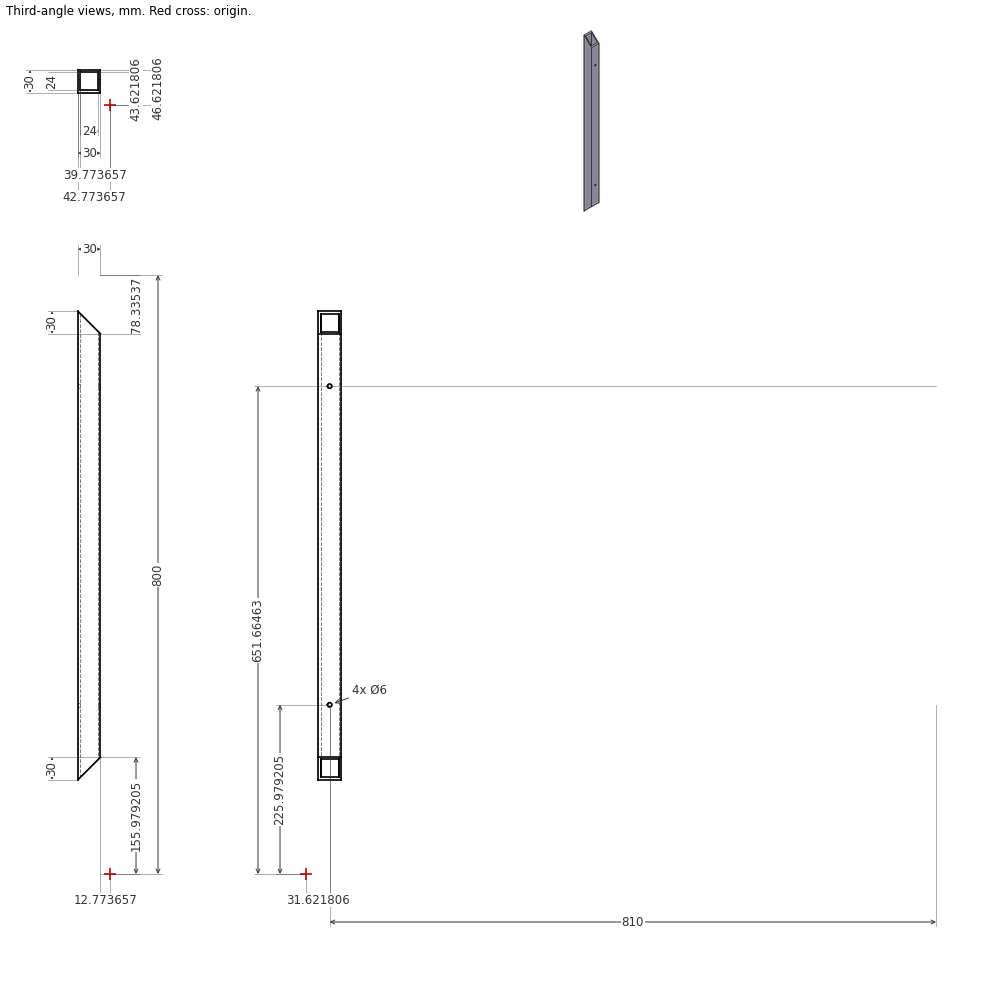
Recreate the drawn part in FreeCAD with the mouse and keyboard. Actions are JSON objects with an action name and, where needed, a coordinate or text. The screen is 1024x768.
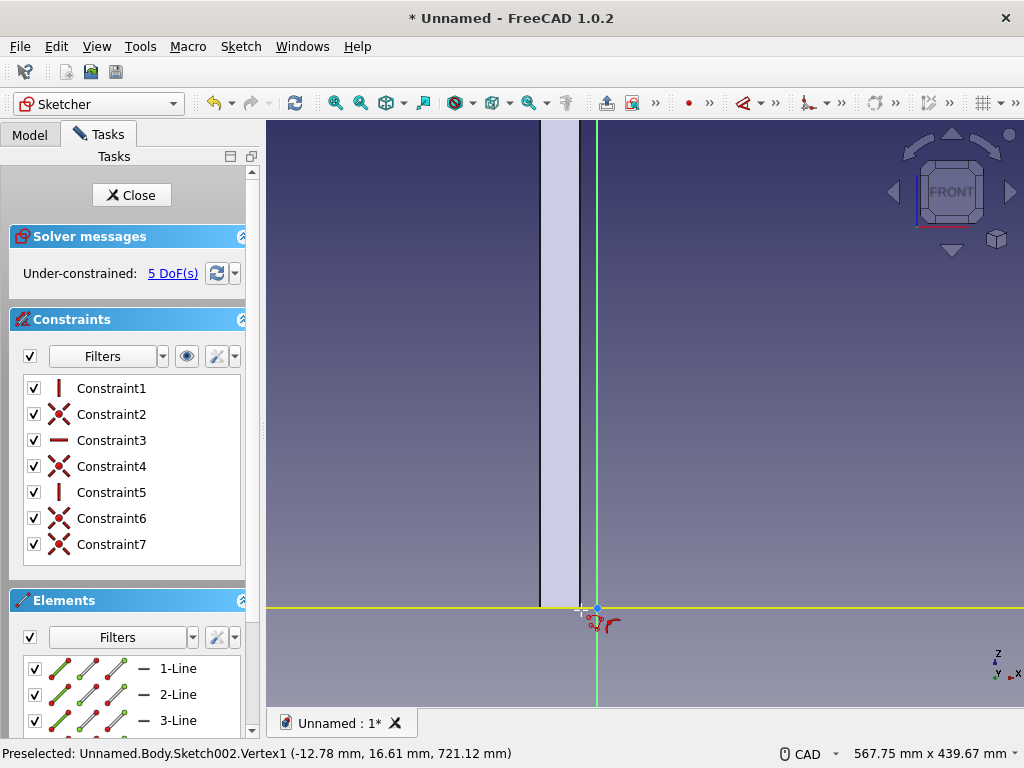
{"action": "left_click", "coordinate": [580, 608]}
{"action": "left_click", "coordinate": [580, 400]}
{"action": "left_click", "coordinate": [540, 440]}
{"action": "left_click", "coordinate": [540, 599]}
{"action": "left_click", "coordinate": [580, 608]}
{"action": "key", "text": "Escape"}
{"action": "key", "text": "Escape"}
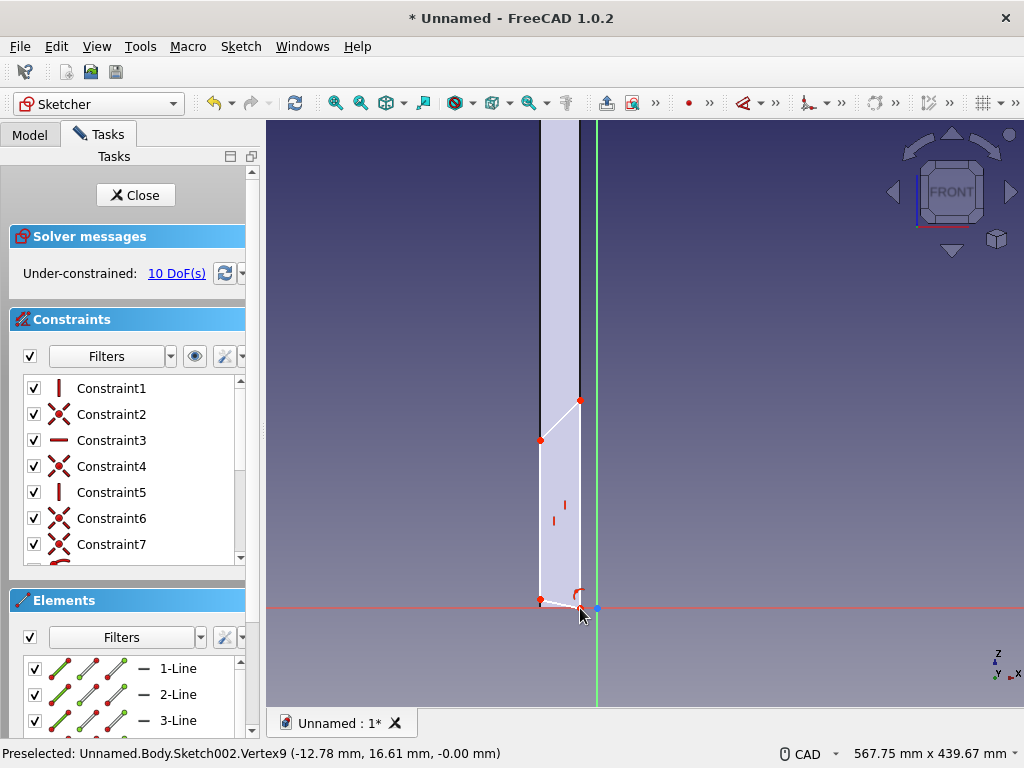
{"action": "left_click", "coordinate": [568, 606]}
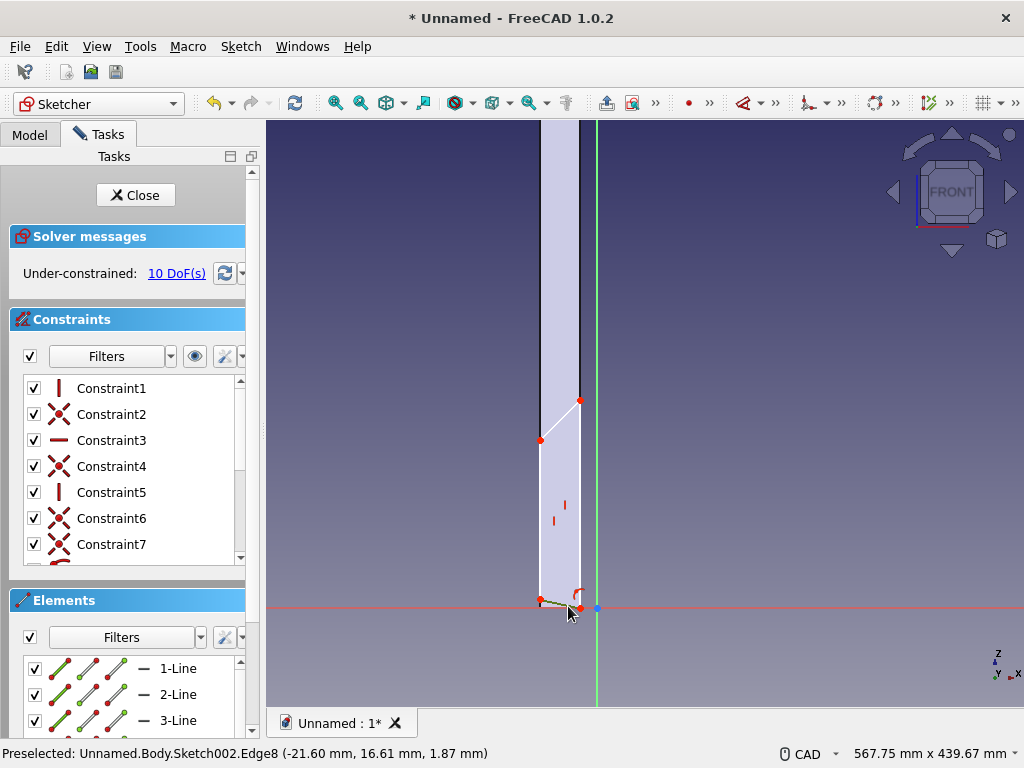
{"action": "key", "text": "h"}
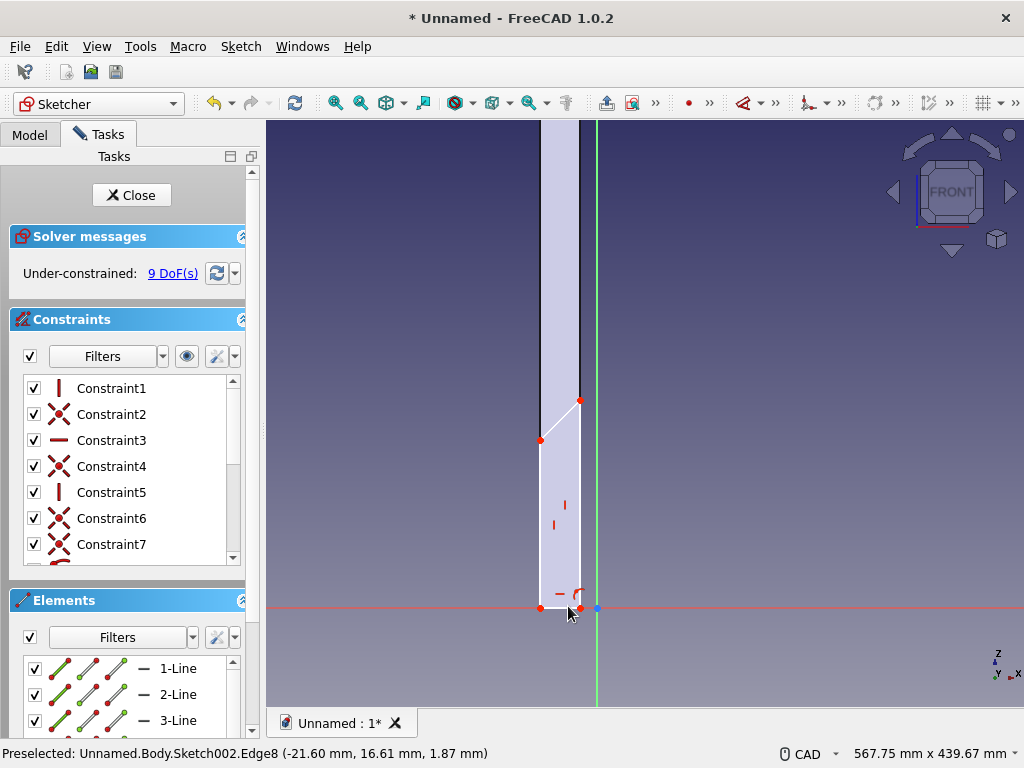
{"action": "key", "text": "d"}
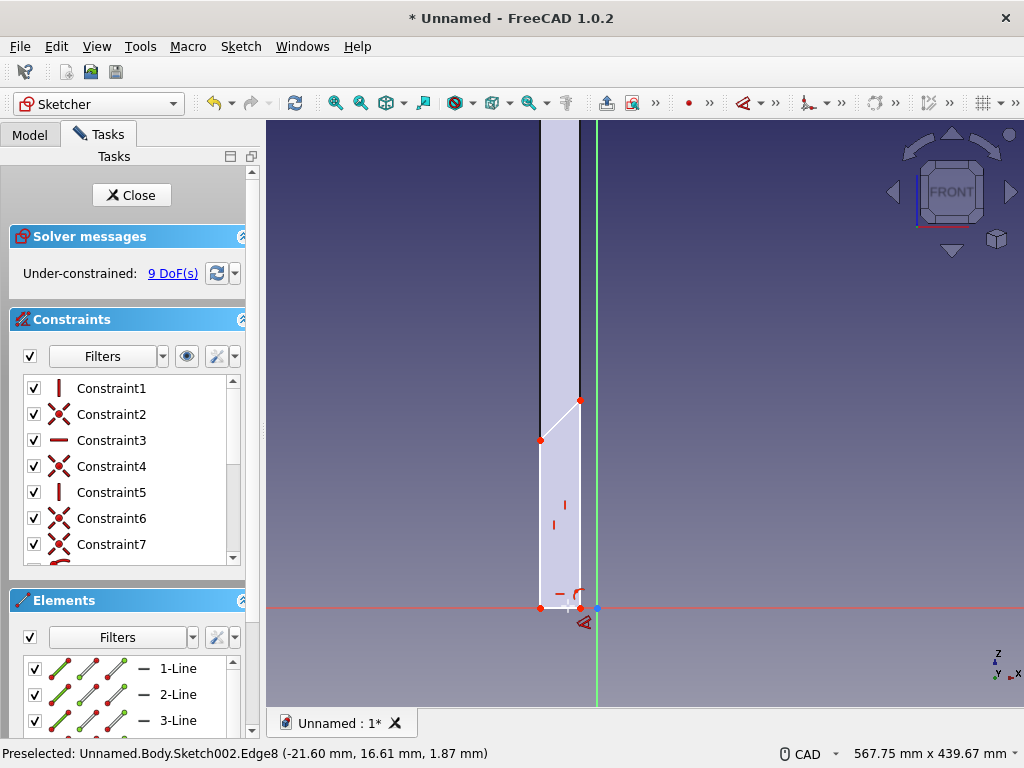
{"action": "scroll", "coordinate": [581, 611], "scroll_direction": "down", "scroll_amount": 5}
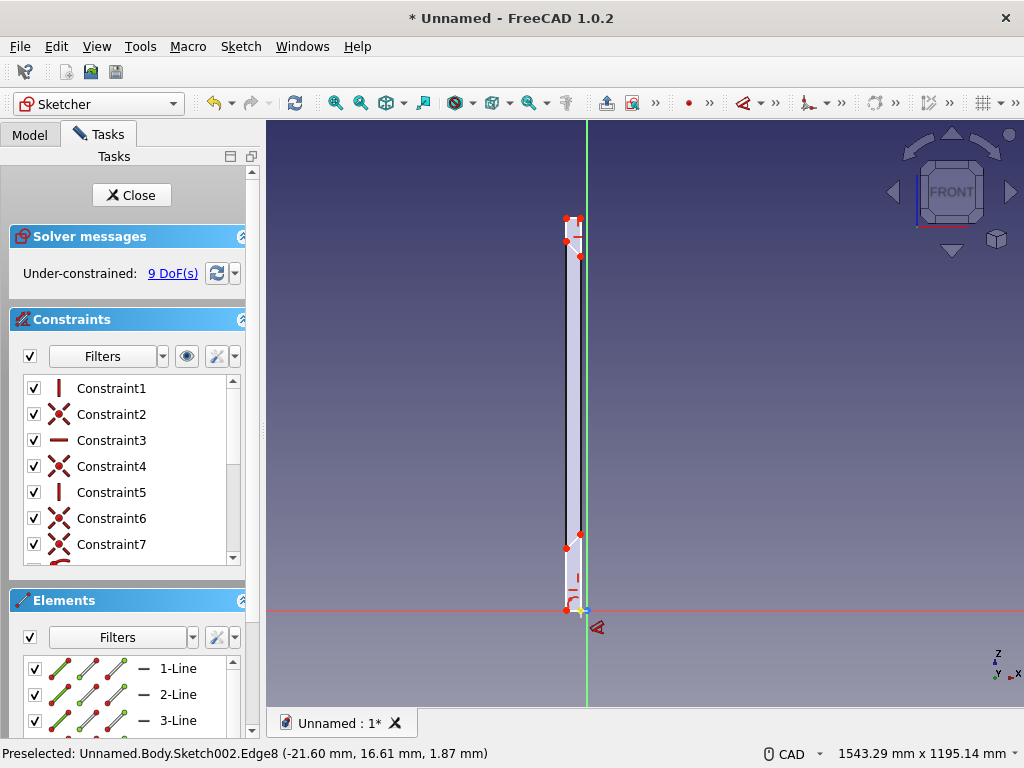
{"action": "scroll", "coordinate": [576, 218], "scroll_direction": "up", "scroll_amount": 6}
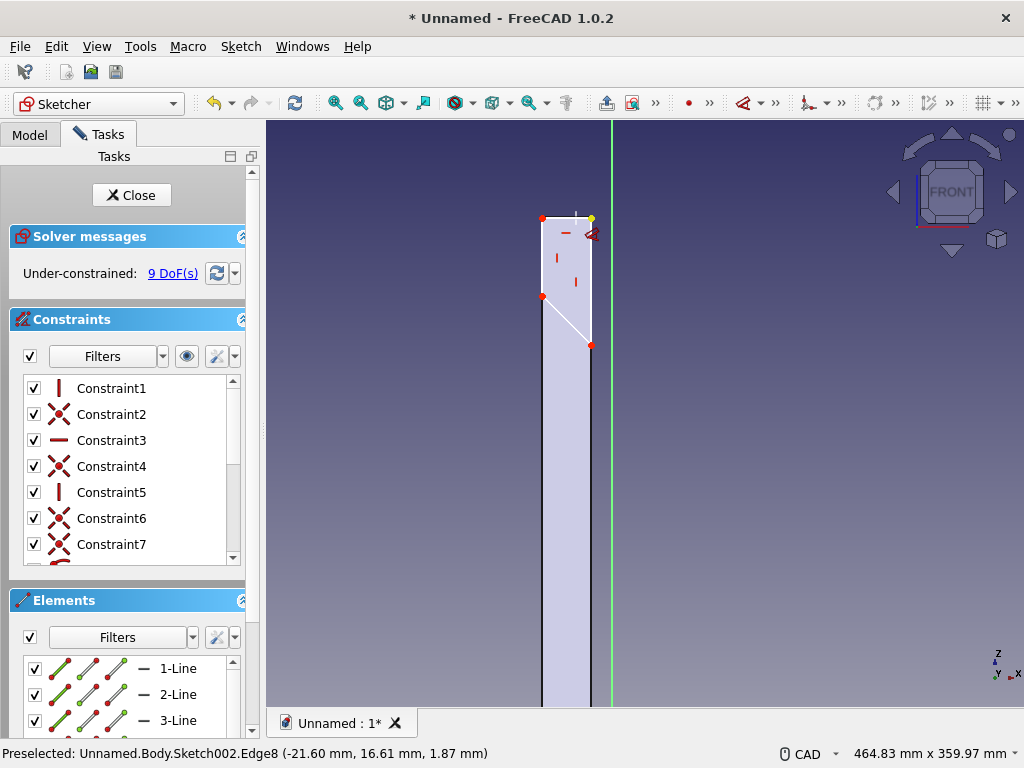
{"action": "left_click", "coordinate": [577, 218]}
{"action": "left_click", "coordinate": [567, 184]}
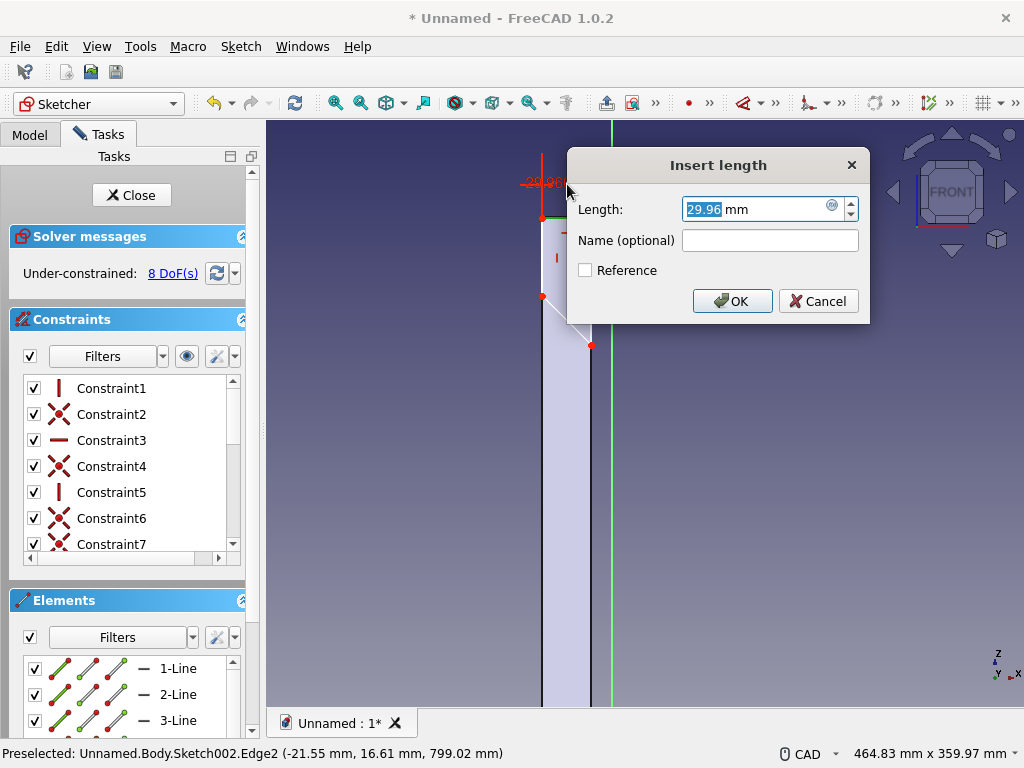
{"action": "type", "text": "30"}
{"action": "key", "text": "Return"}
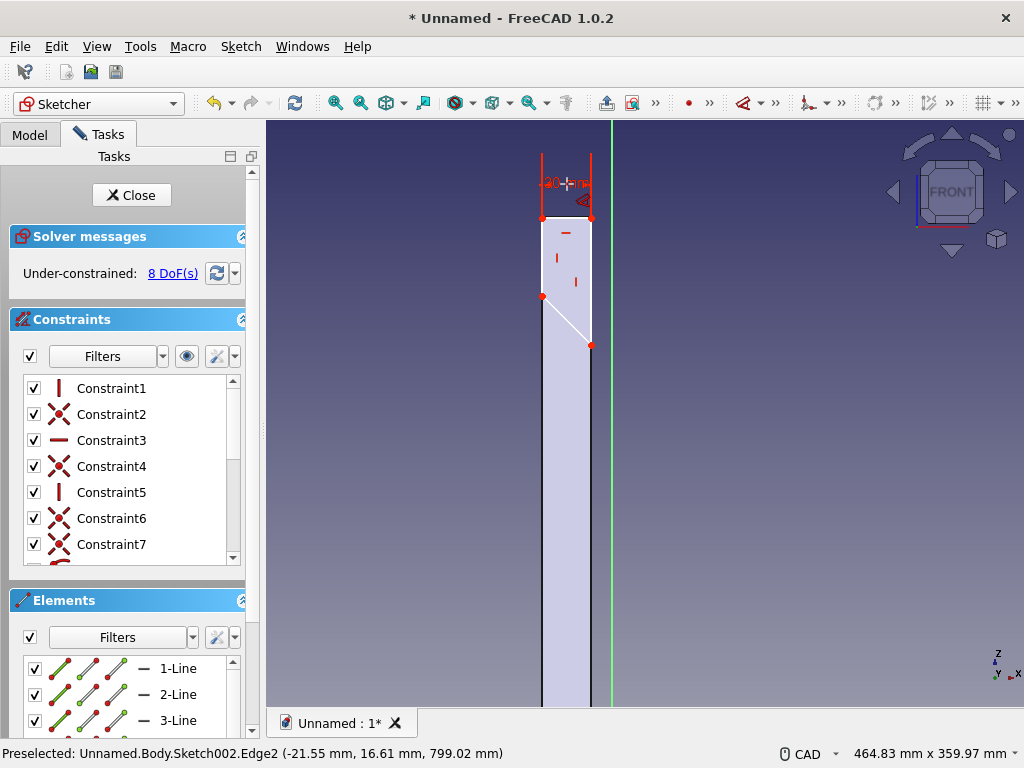
{"action": "scroll", "coordinate": [576, 217], "scroll_direction": "down", "scroll_amount": 6}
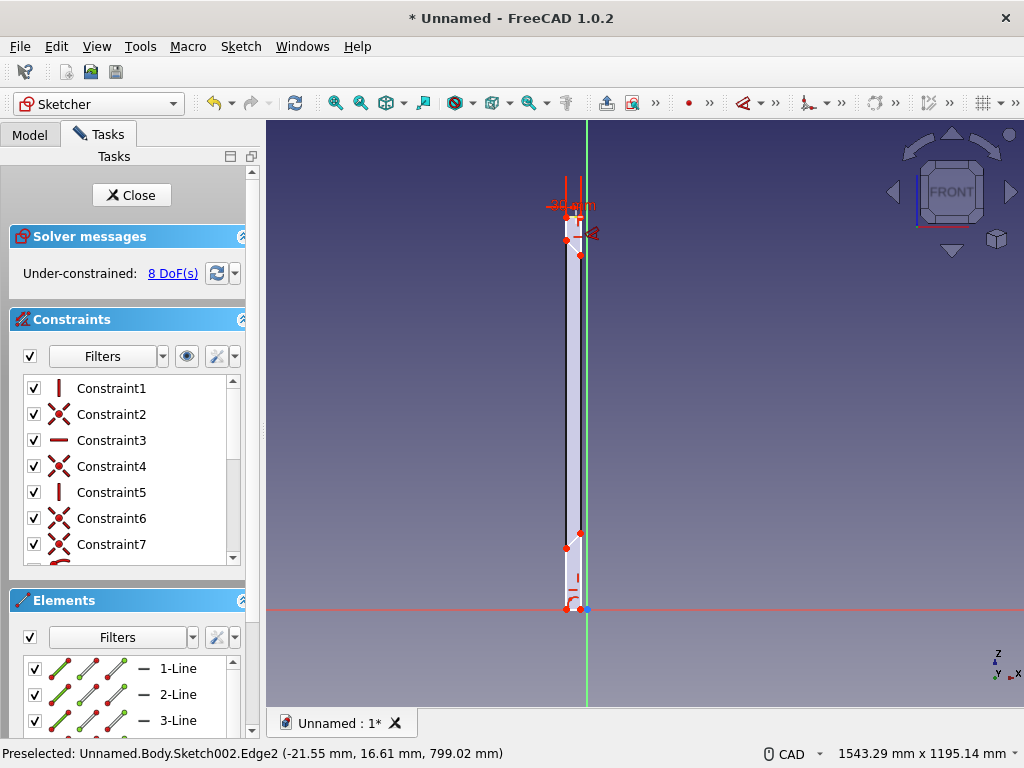
{"action": "scroll", "coordinate": [571, 610], "scroll_direction": "up", "scroll_amount": 6}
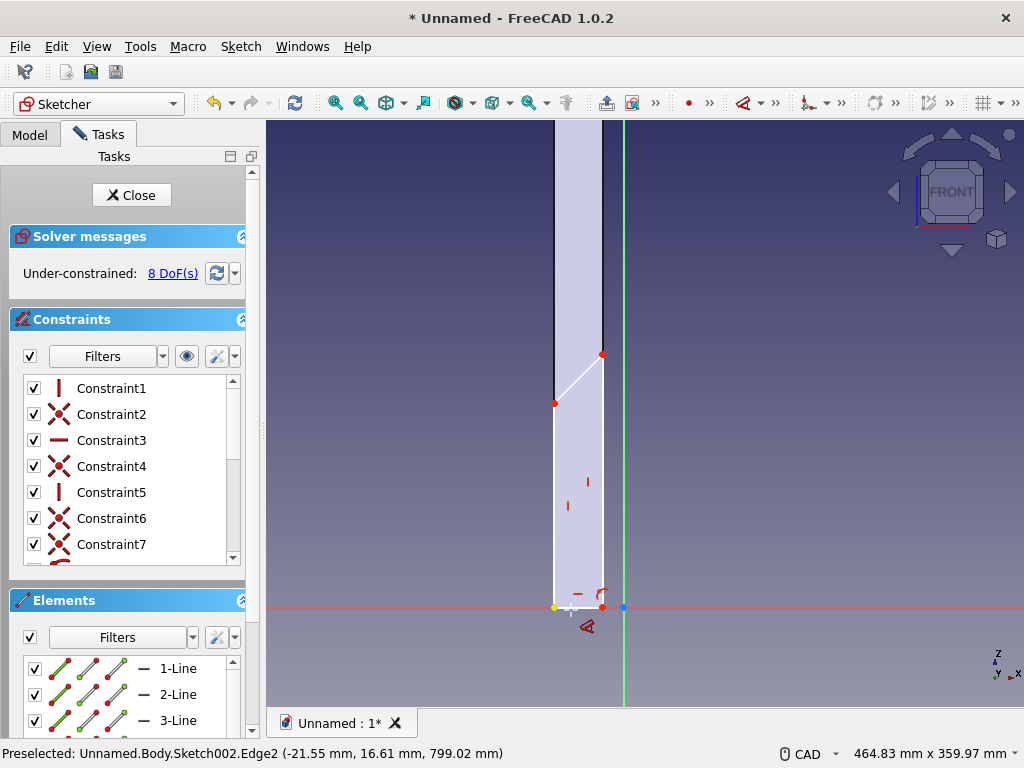
{"action": "left_click", "coordinate": [569, 608]}
{"action": "left_click", "coordinate": [578, 642]}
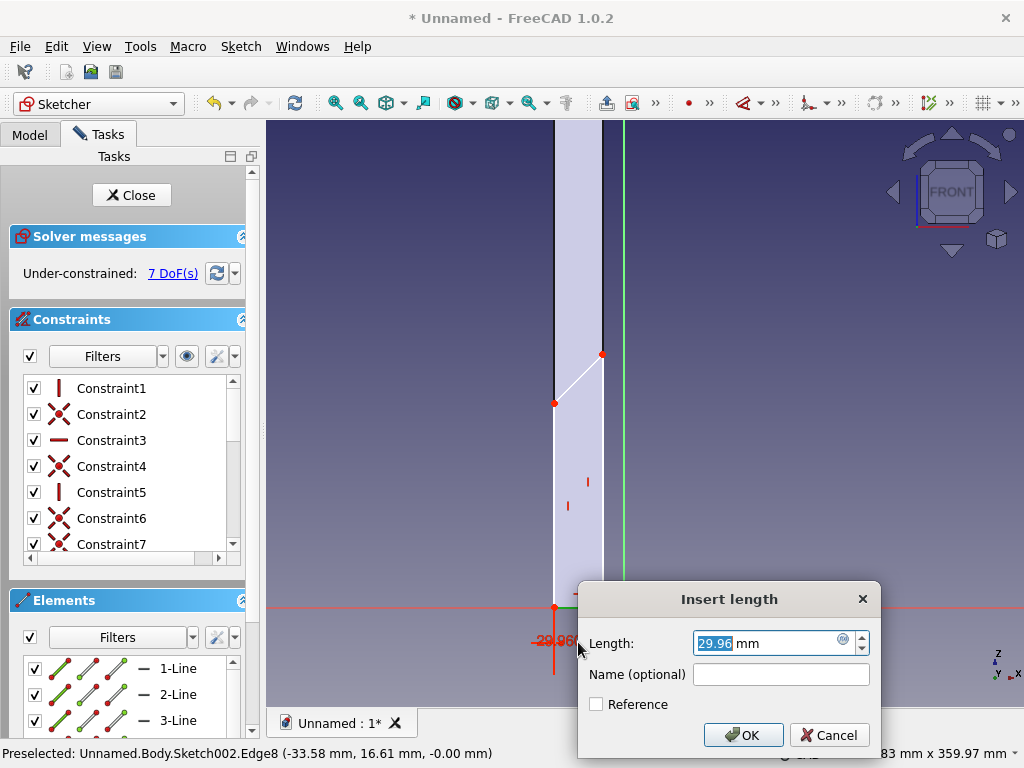
{"action": "type", "text": "30"}
{"action": "key", "text": "Return"}